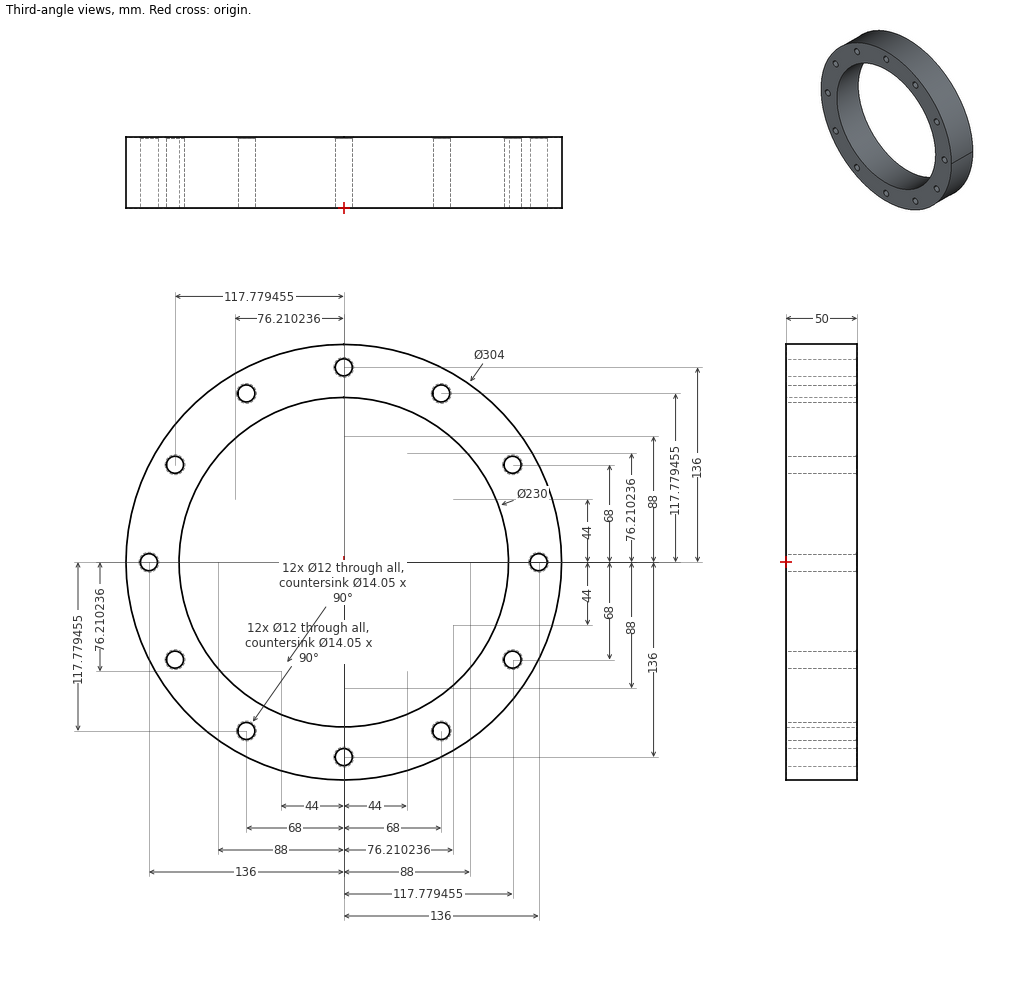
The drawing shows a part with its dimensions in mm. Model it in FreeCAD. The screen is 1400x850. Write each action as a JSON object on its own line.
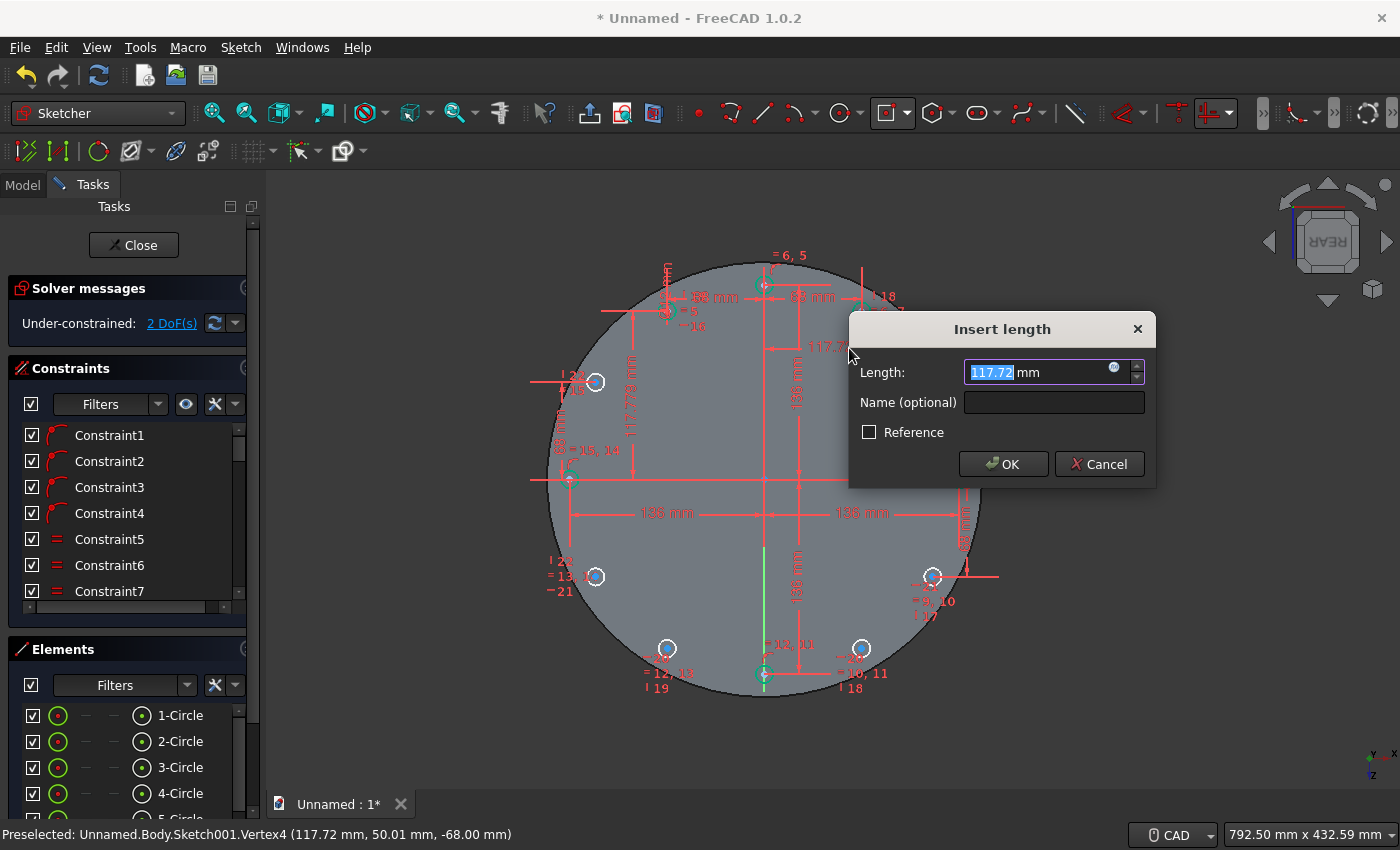
{"action": "type", "text": "117.779455"}
{"action": "key", "text": "Return"}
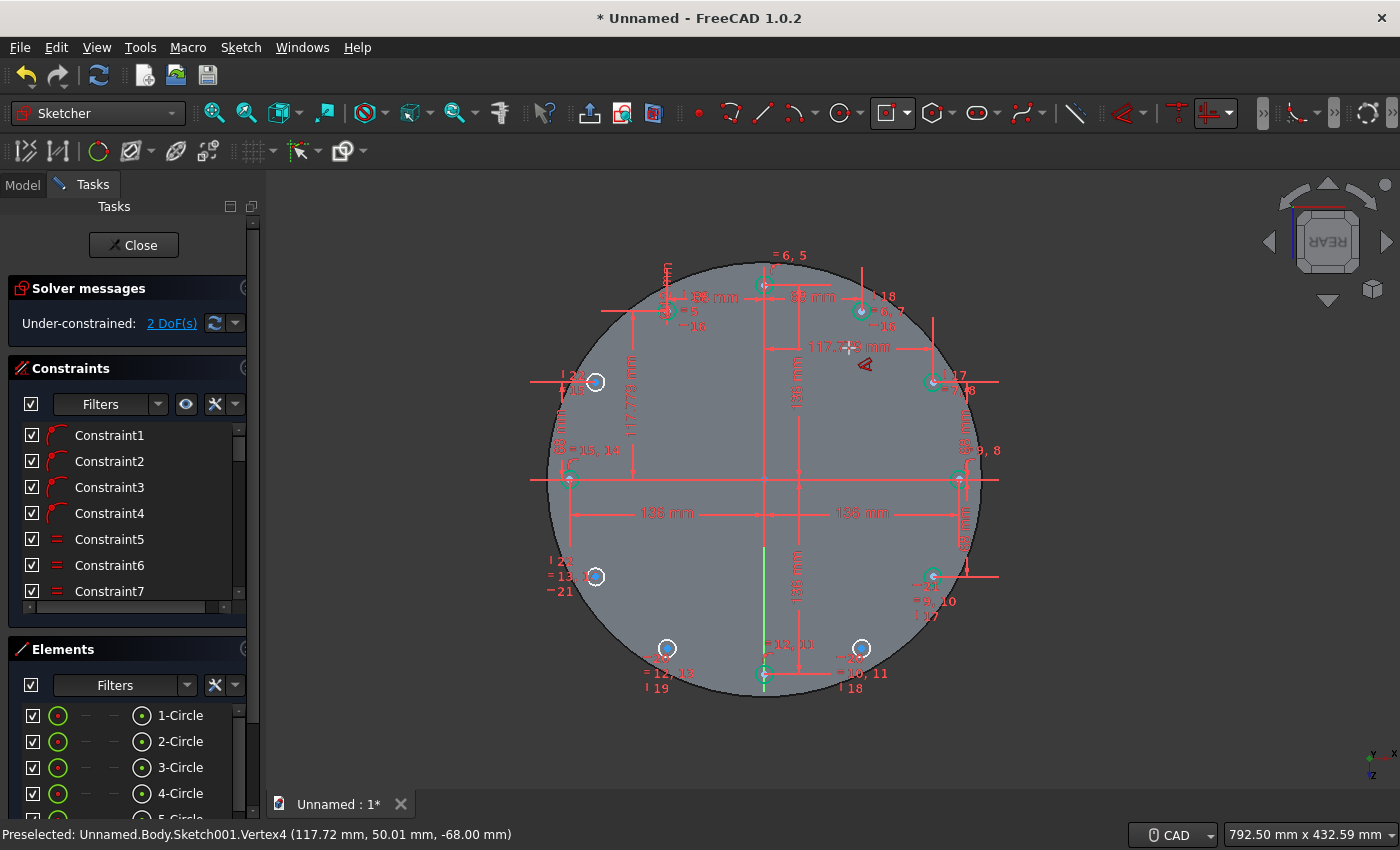
{"action": "left_click", "coordinate": [862, 649]}
{"action": "left_click", "coordinate": [896, 564]}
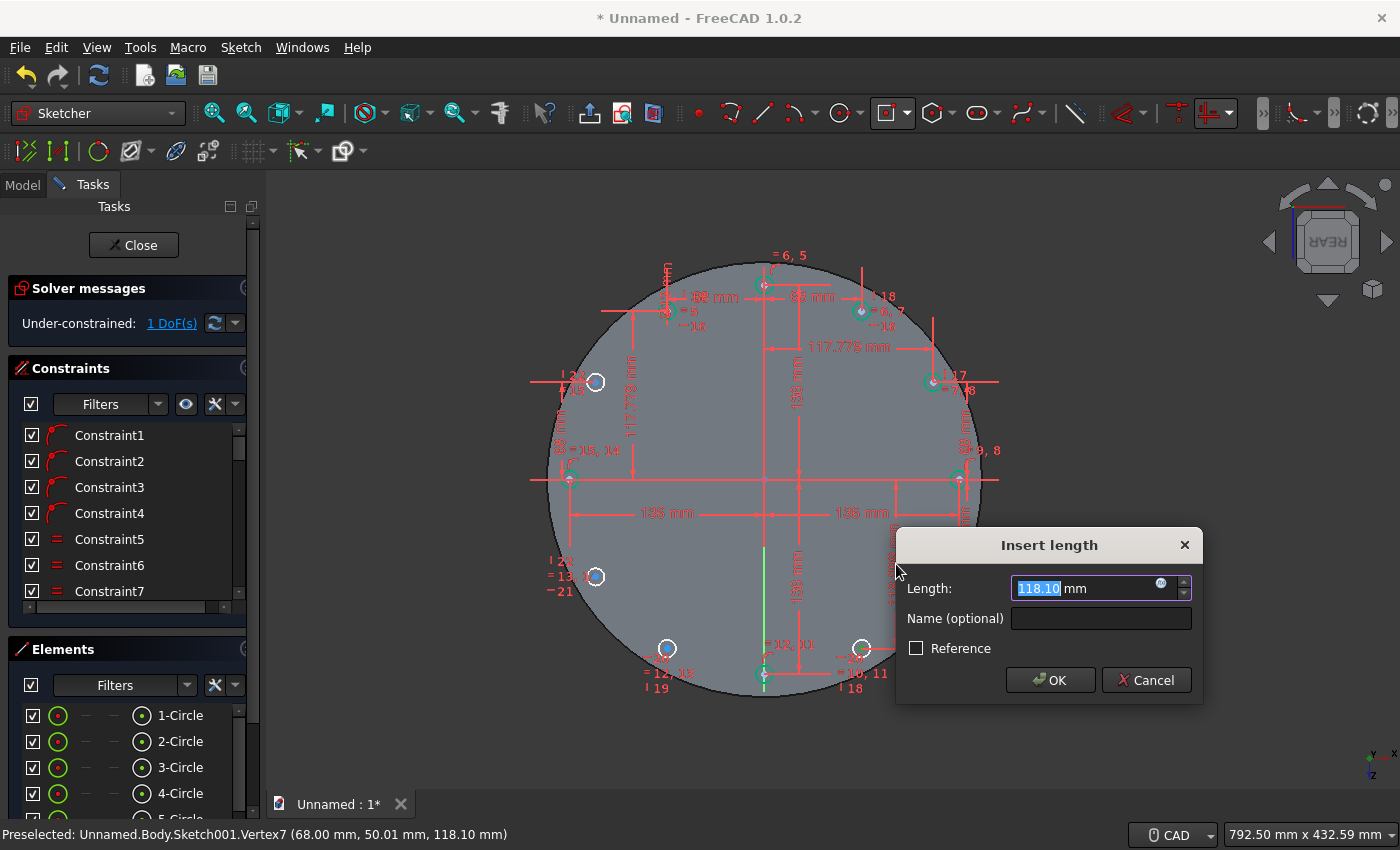
{"action": "type", "text": "117.779455"}
{"action": "key", "text": "Return"}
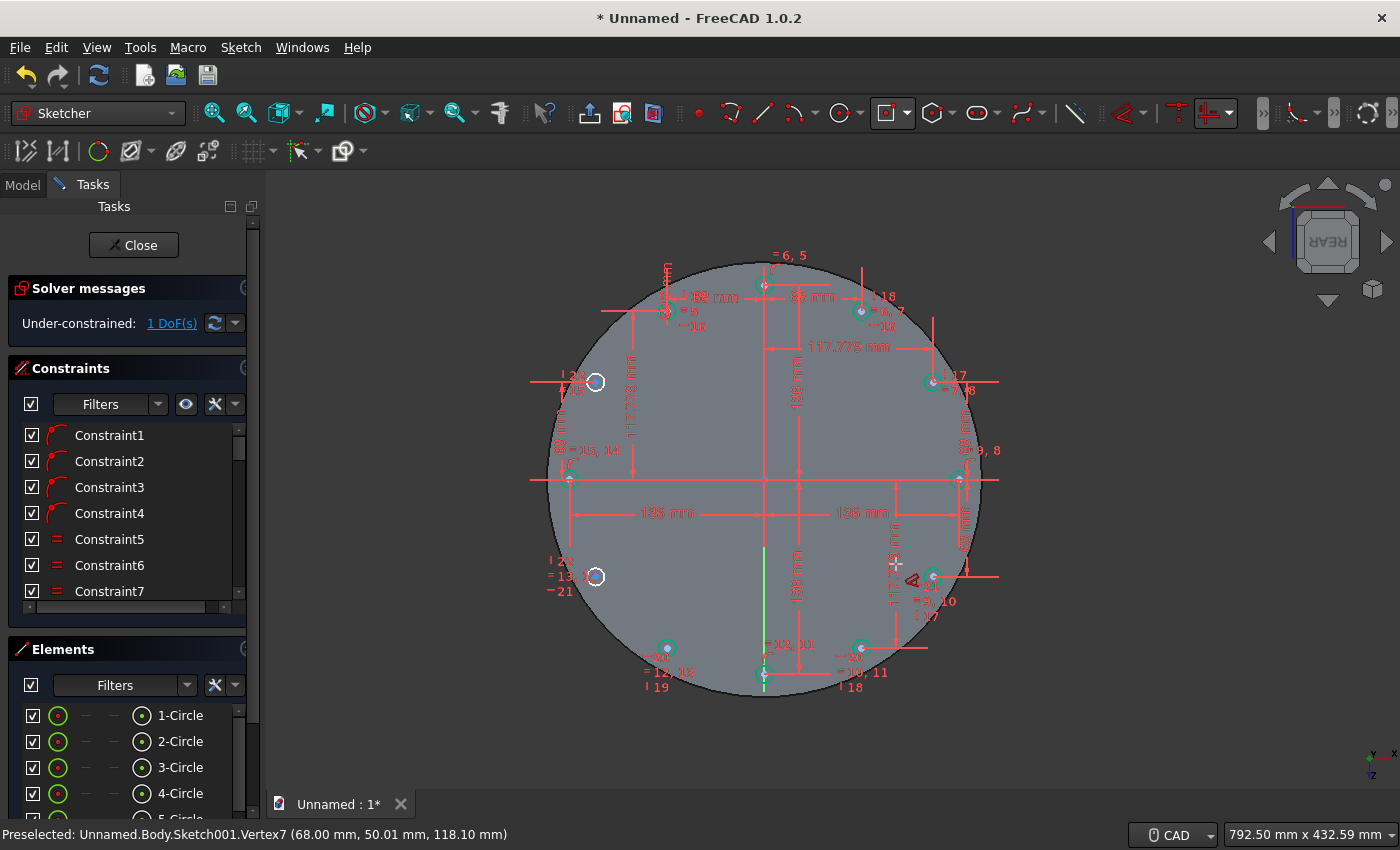
{"action": "left_click", "coordinate": [596, 577]}
{"action": "left_click", "coordinate": [680, 611]}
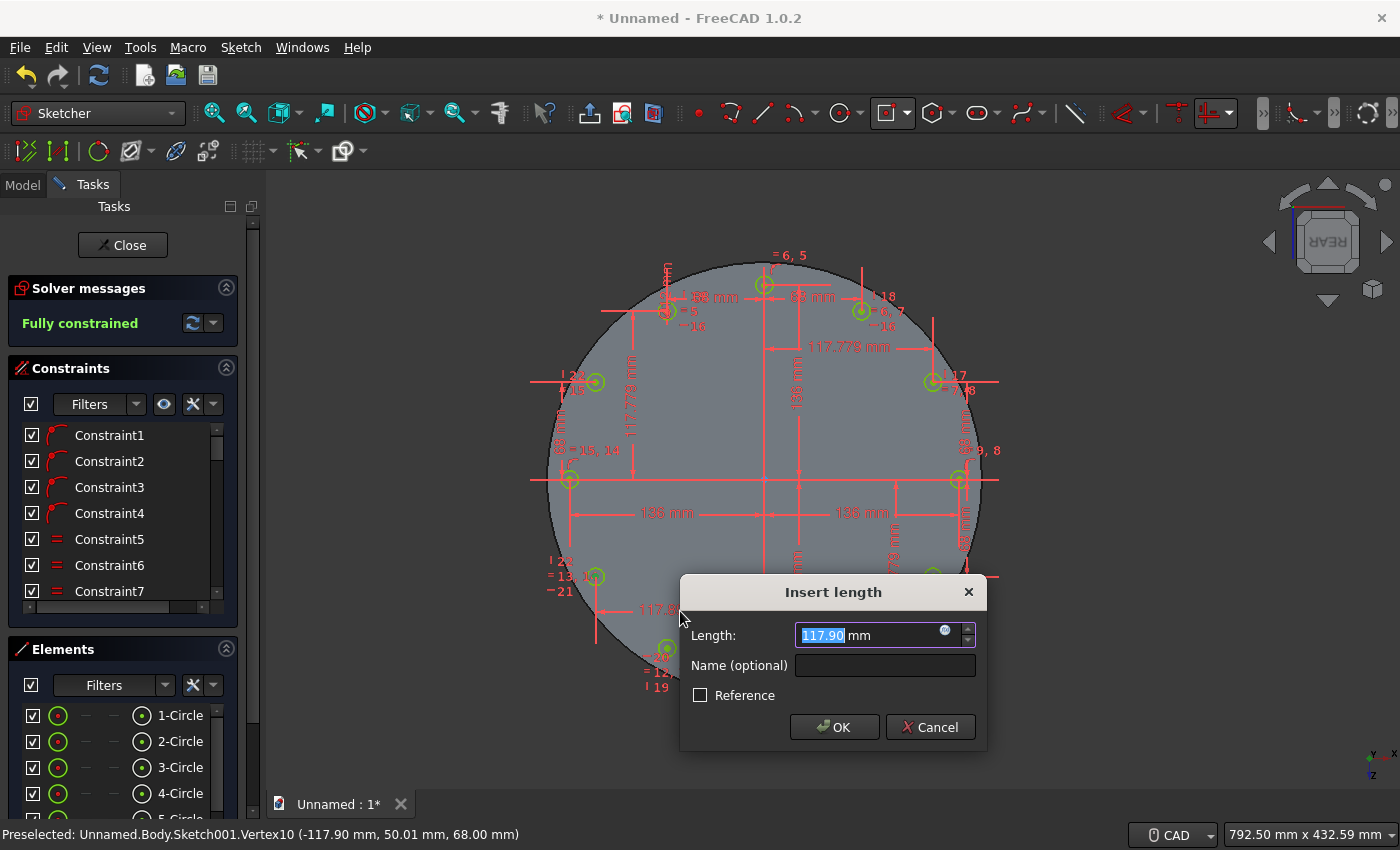
{"action": "type", "text": "117.779455"}
{"action": "key", "text": "Return"}
{"action": "key", "text": "Escape"}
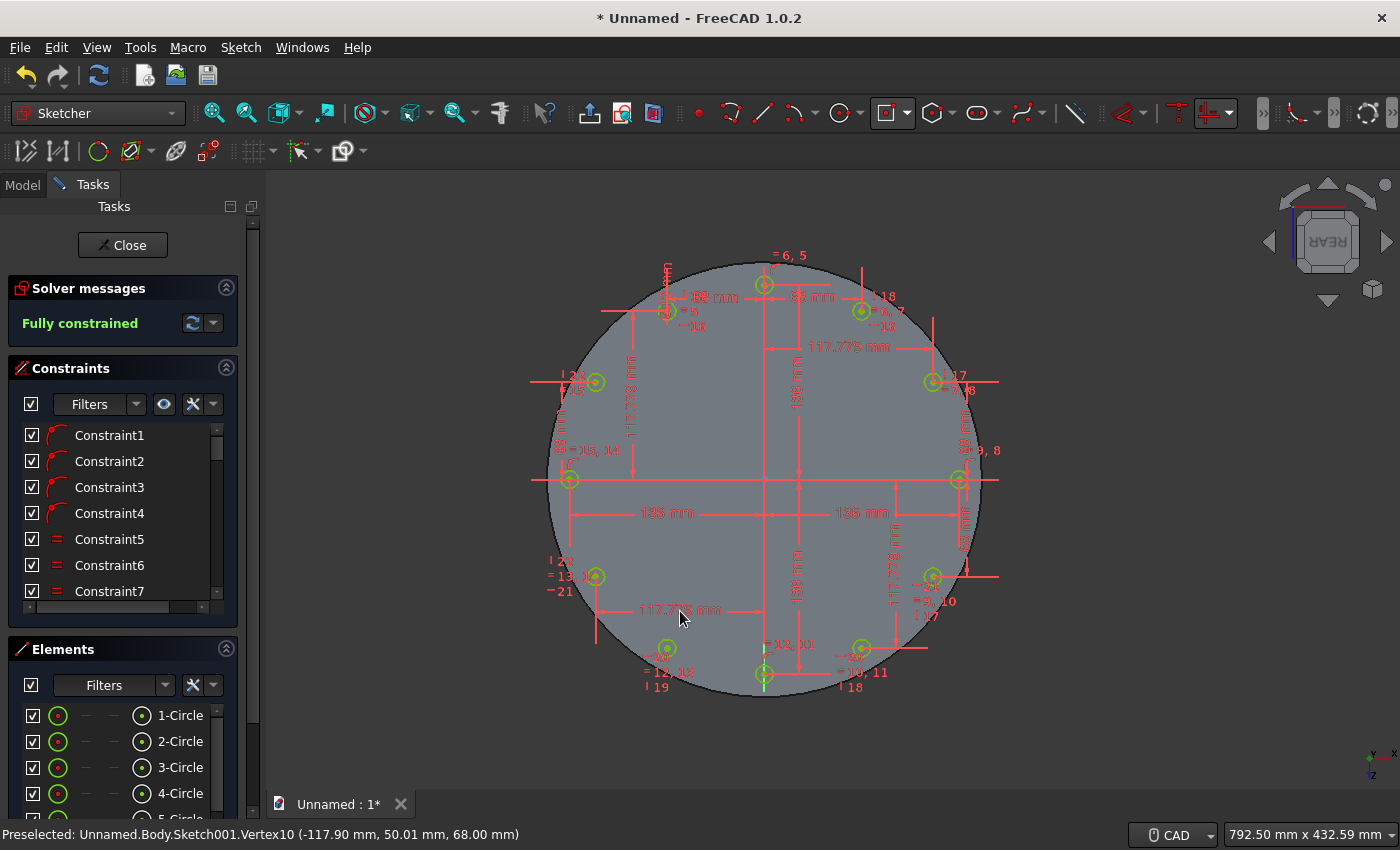
{"action": "left_click", "coordinate": [123, 245]}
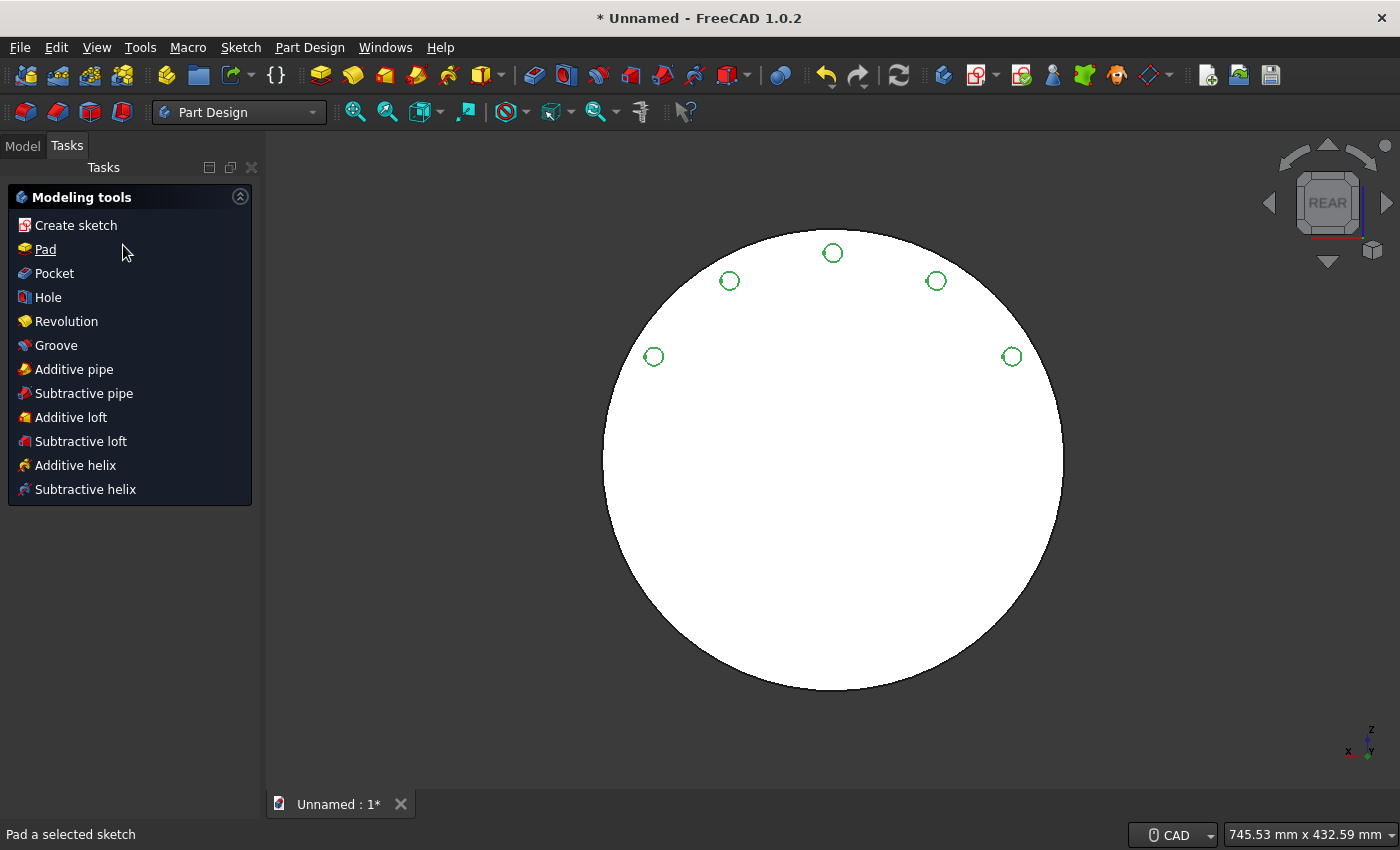
{"action": "left_click", "coordinate": [568, 76]}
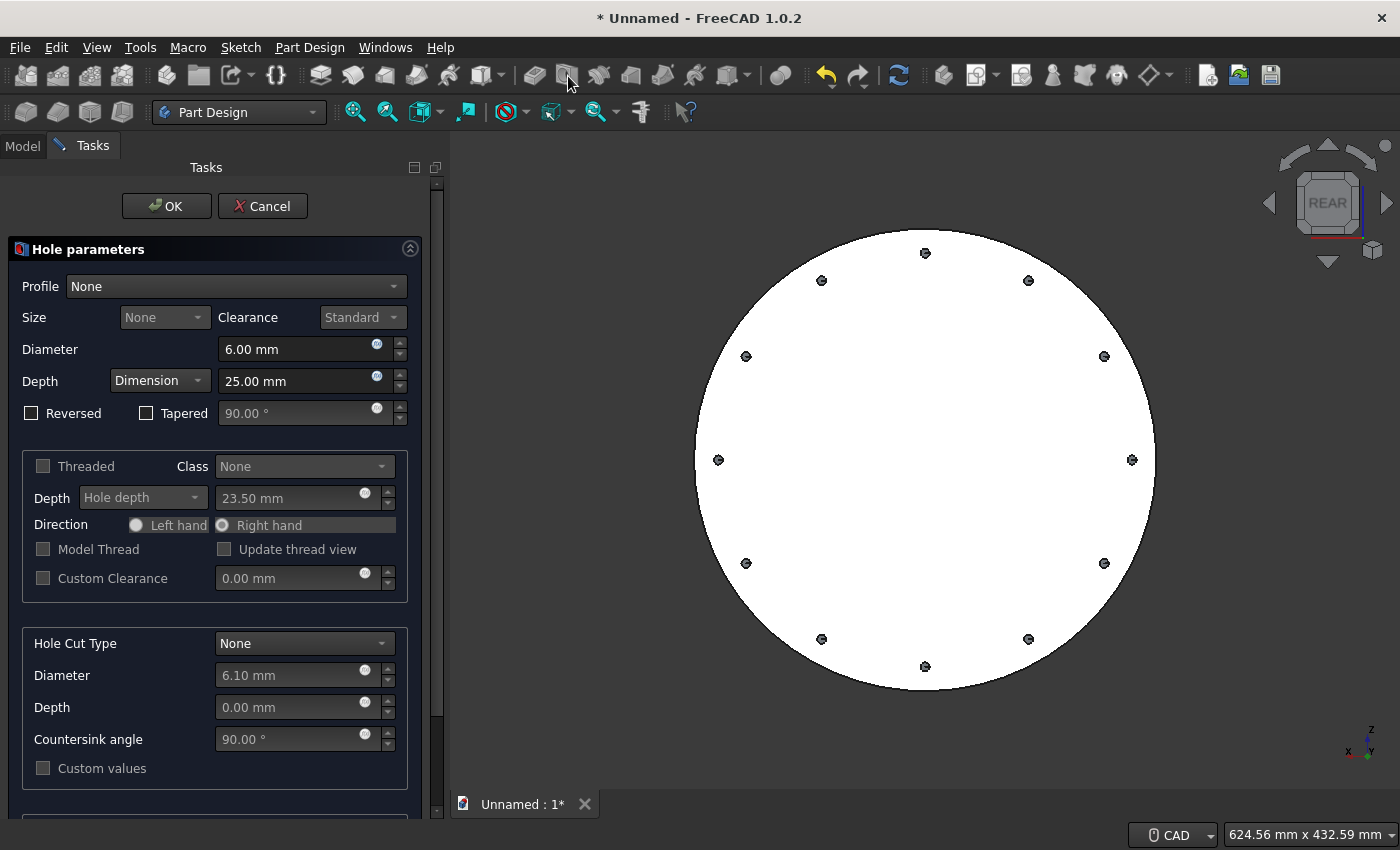
{"action": "triple_click", "coordinate": [305, 349]}